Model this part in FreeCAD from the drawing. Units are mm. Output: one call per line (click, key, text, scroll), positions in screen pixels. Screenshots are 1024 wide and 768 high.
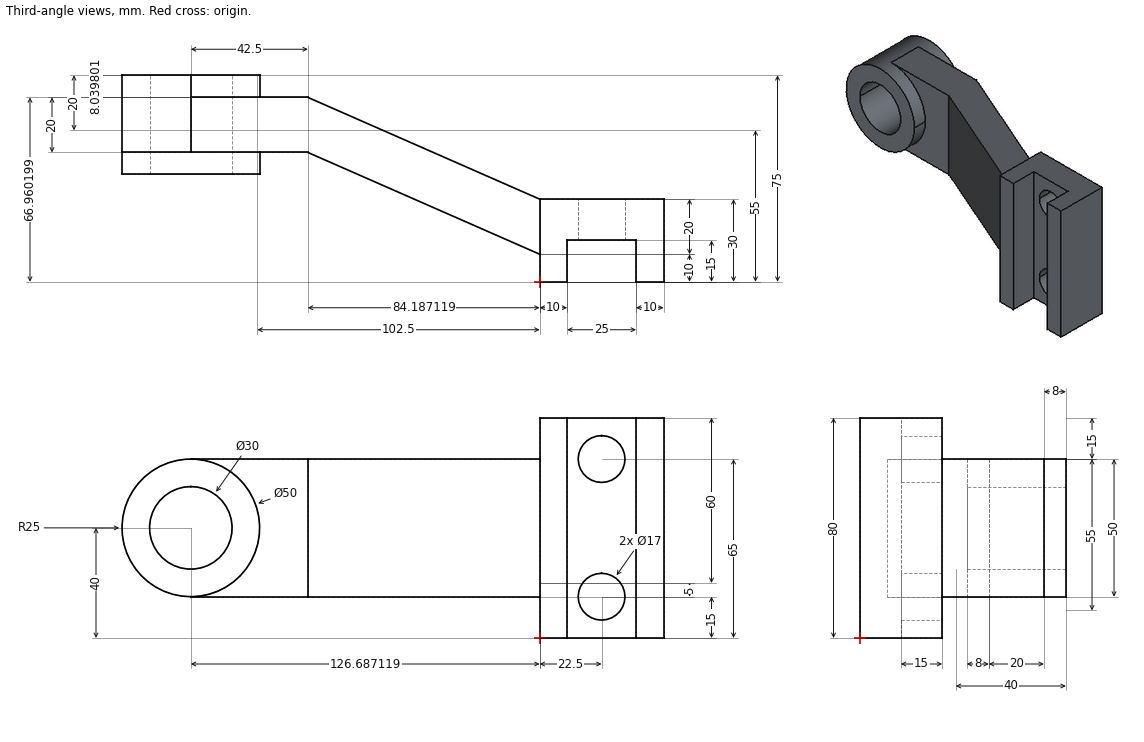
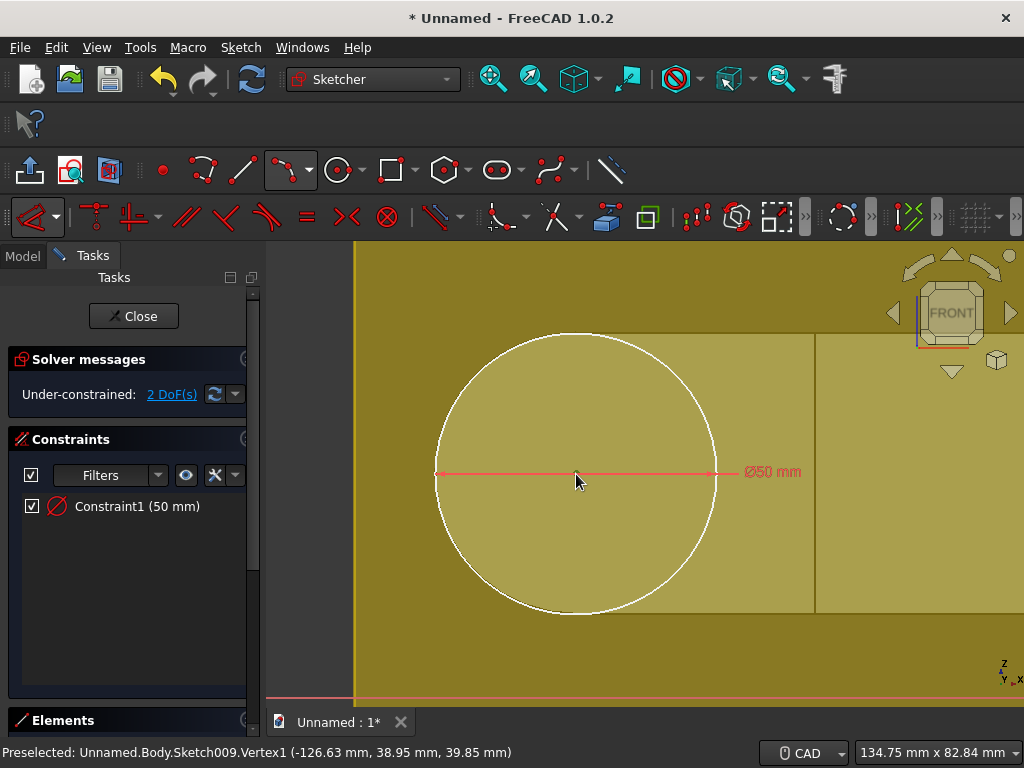
key(i)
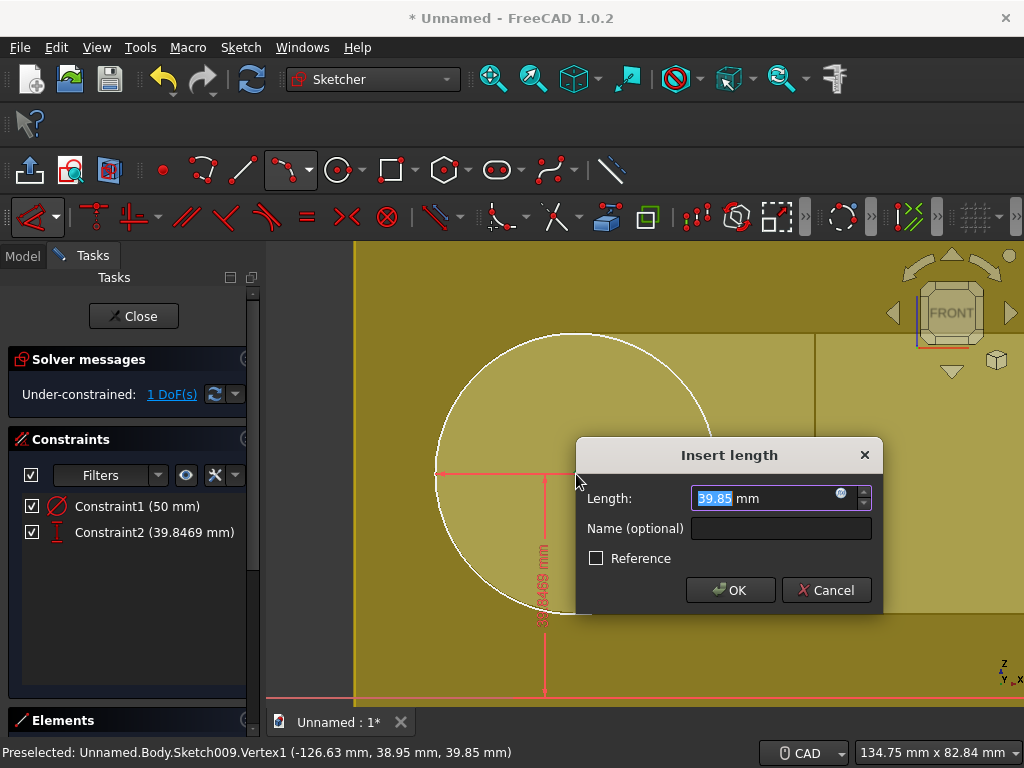
text(40)
key(Return)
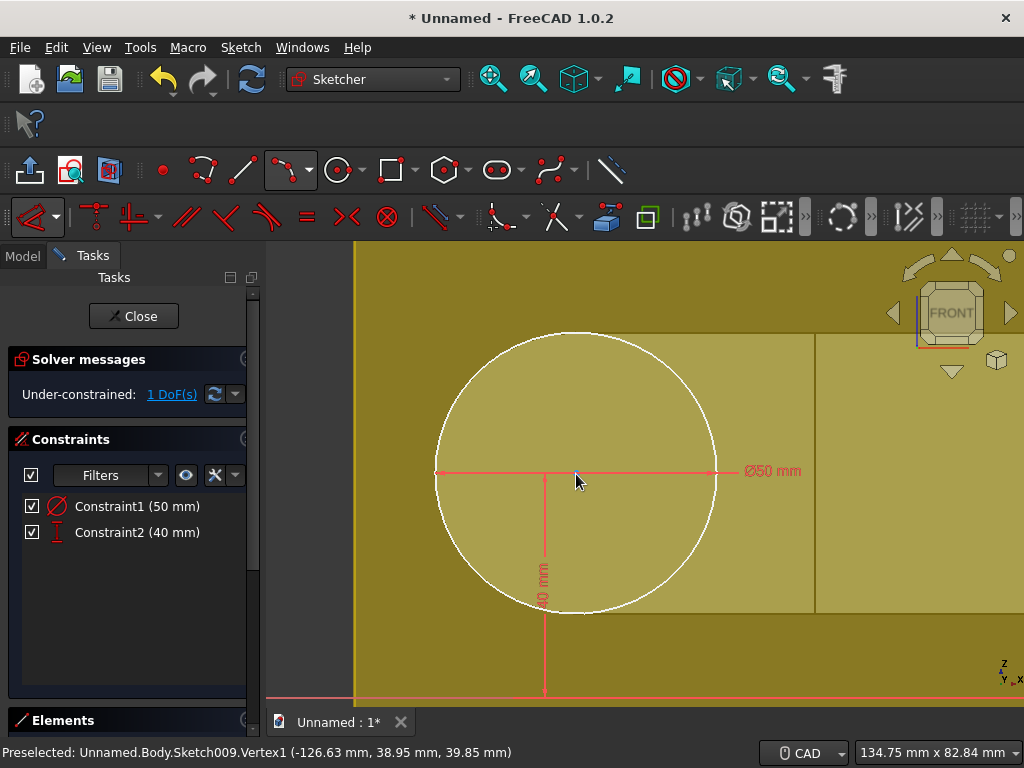
click(576, 473)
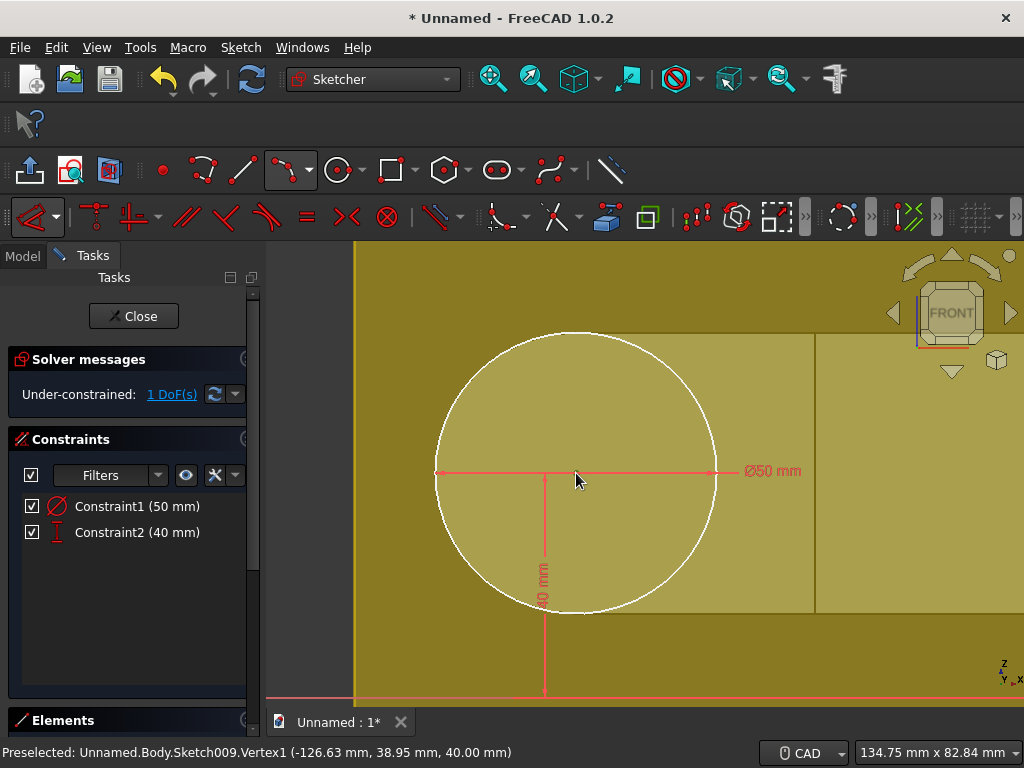
key(l)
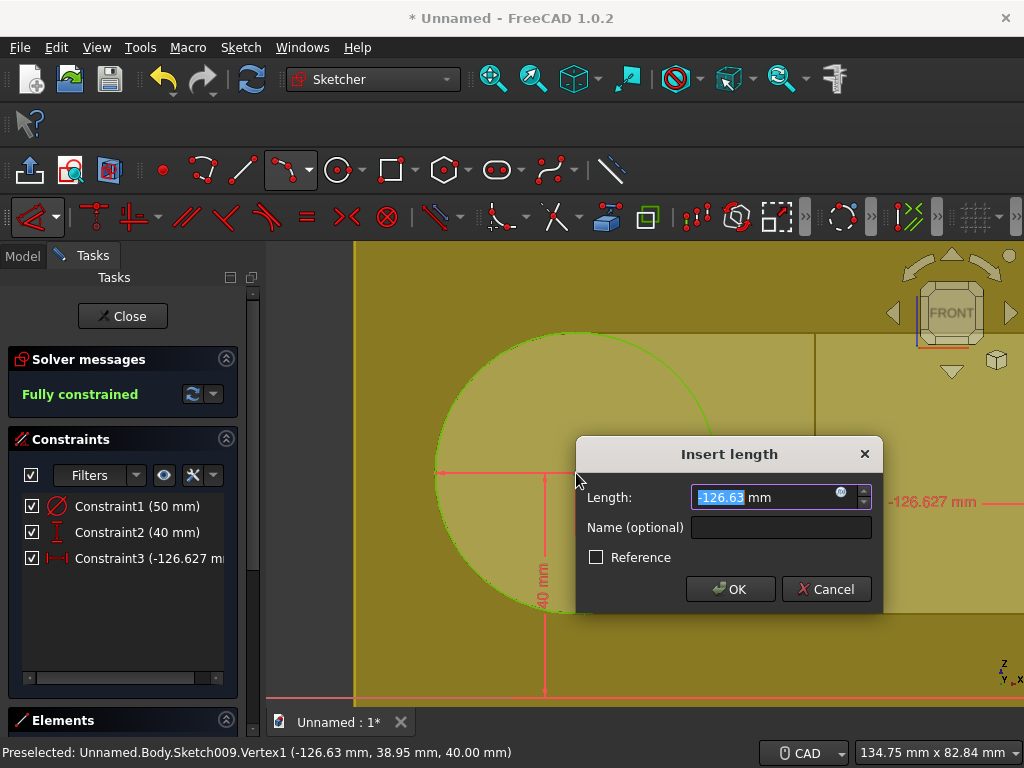
text(-126.687119)
key(Return)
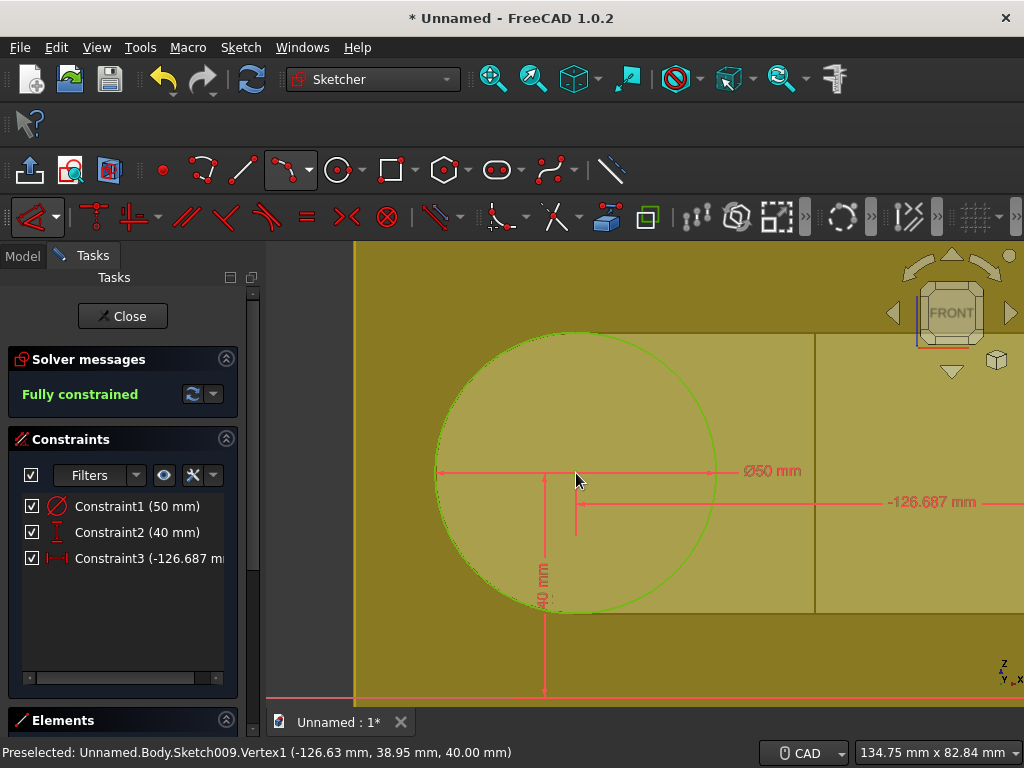
click(123, 316)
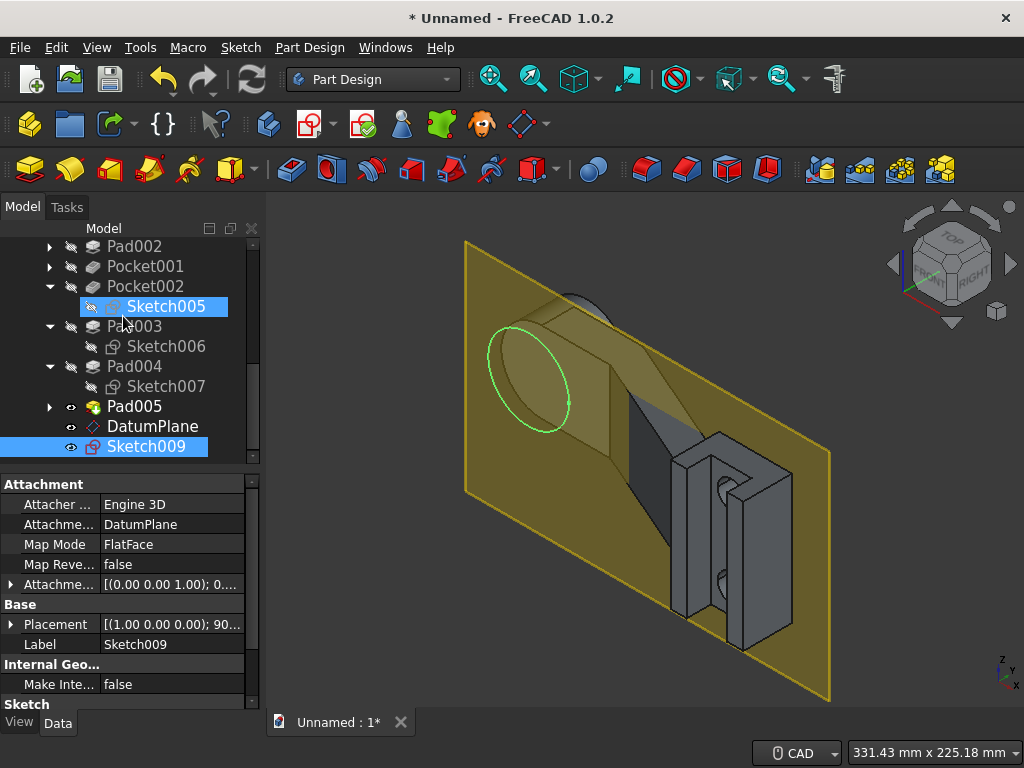
click(30, 170)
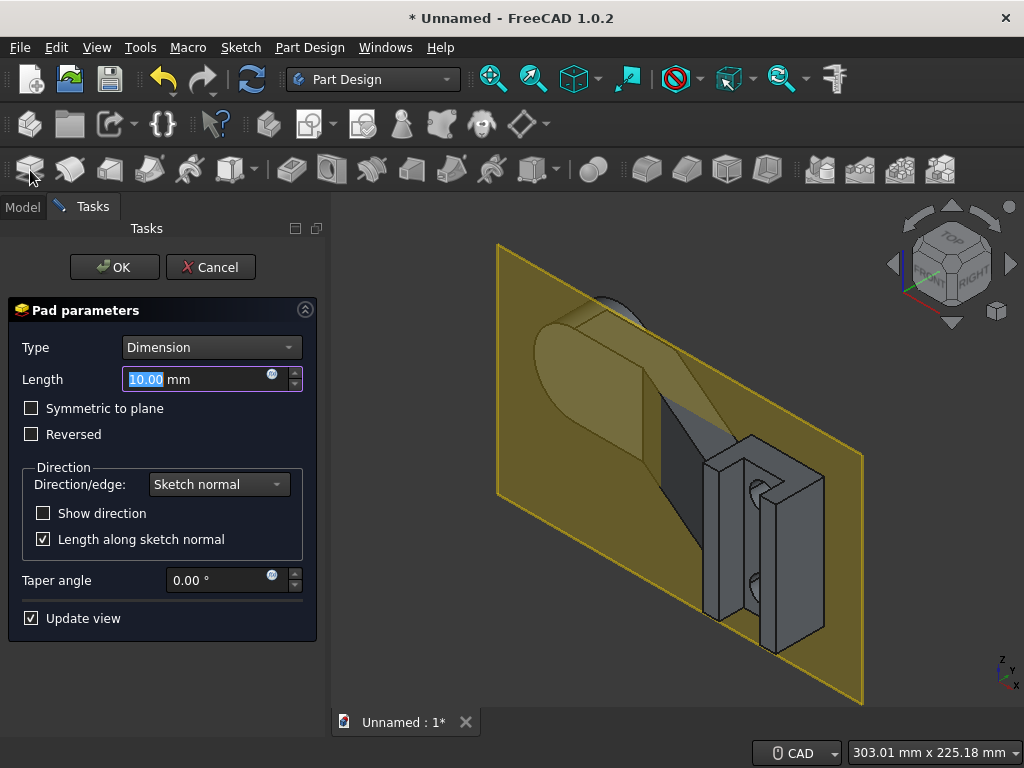
text(8)
key(Tab)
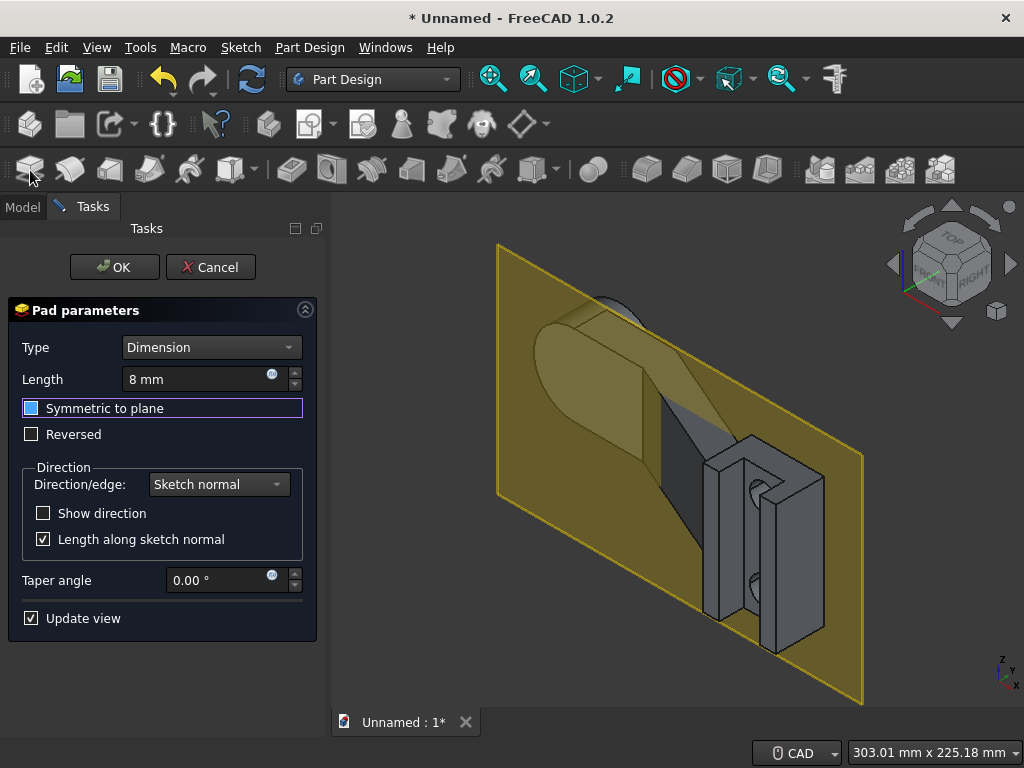
click(30, 434)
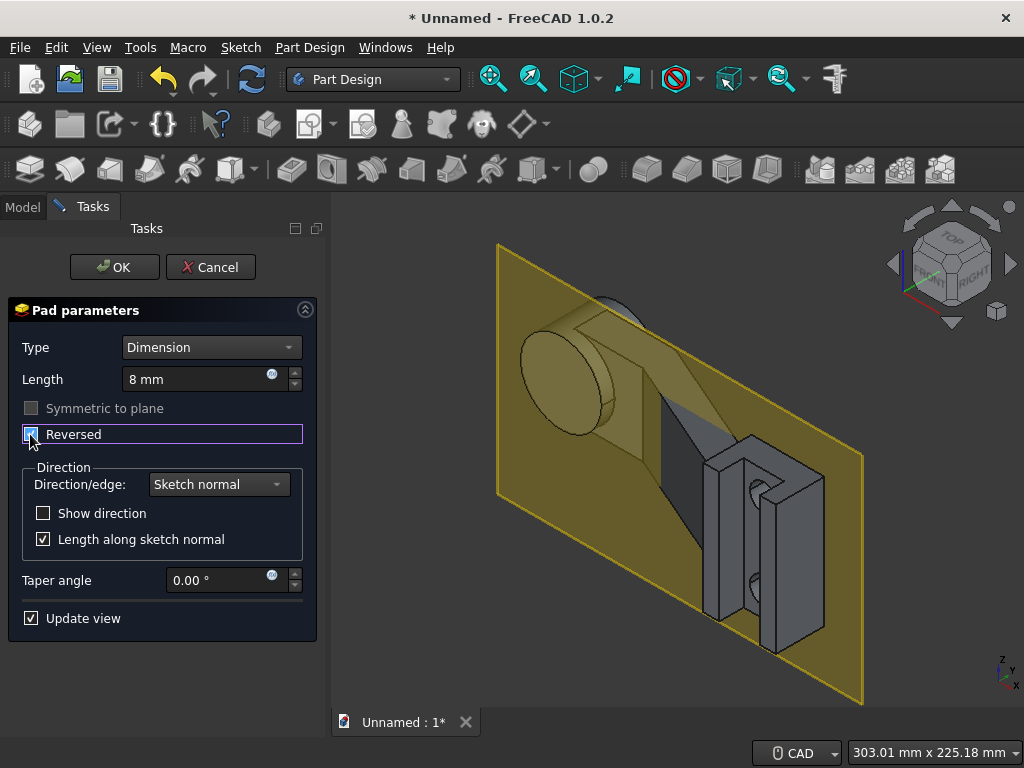
click(115, 267)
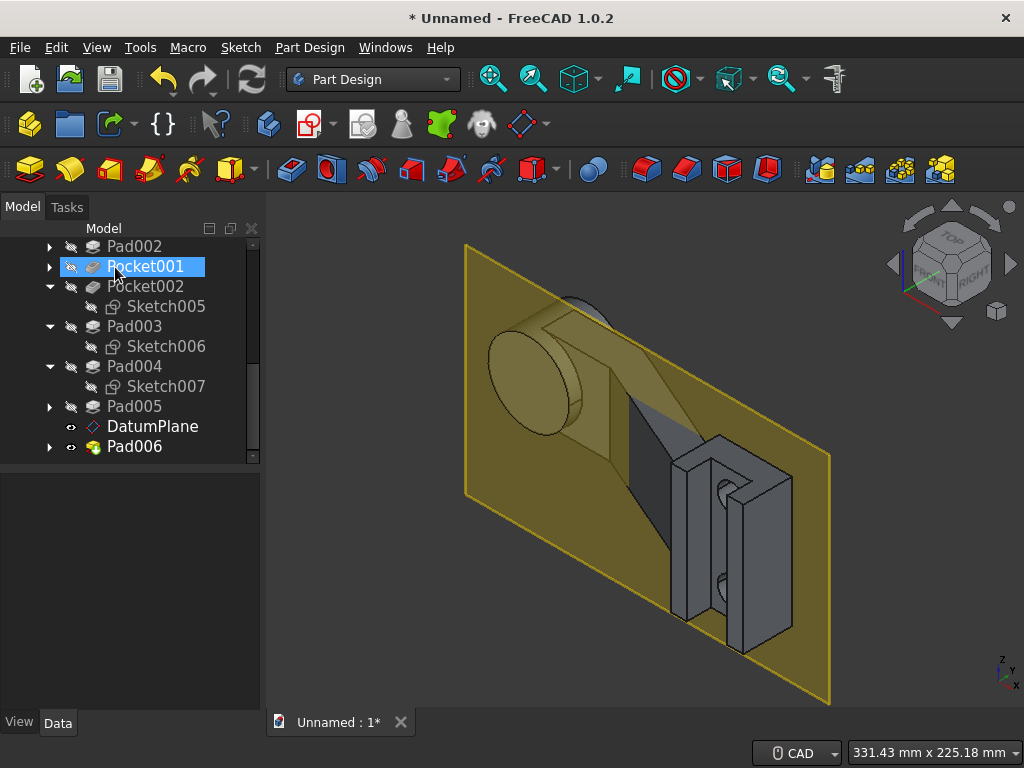
click(116, 427)
key(space)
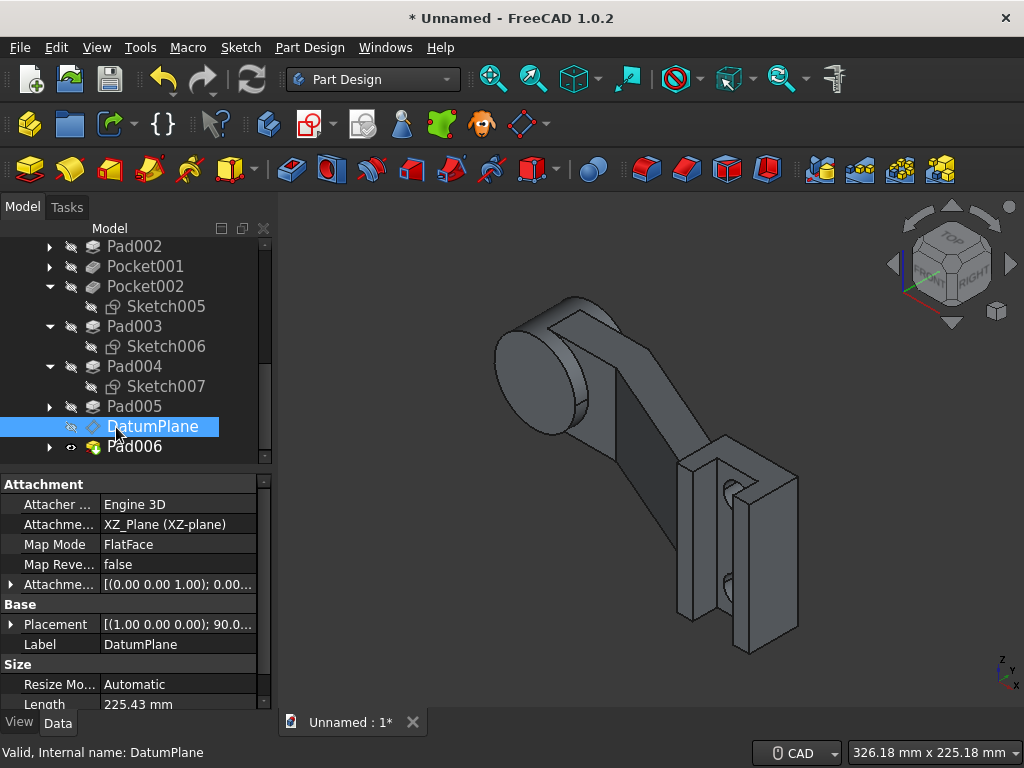
key(4)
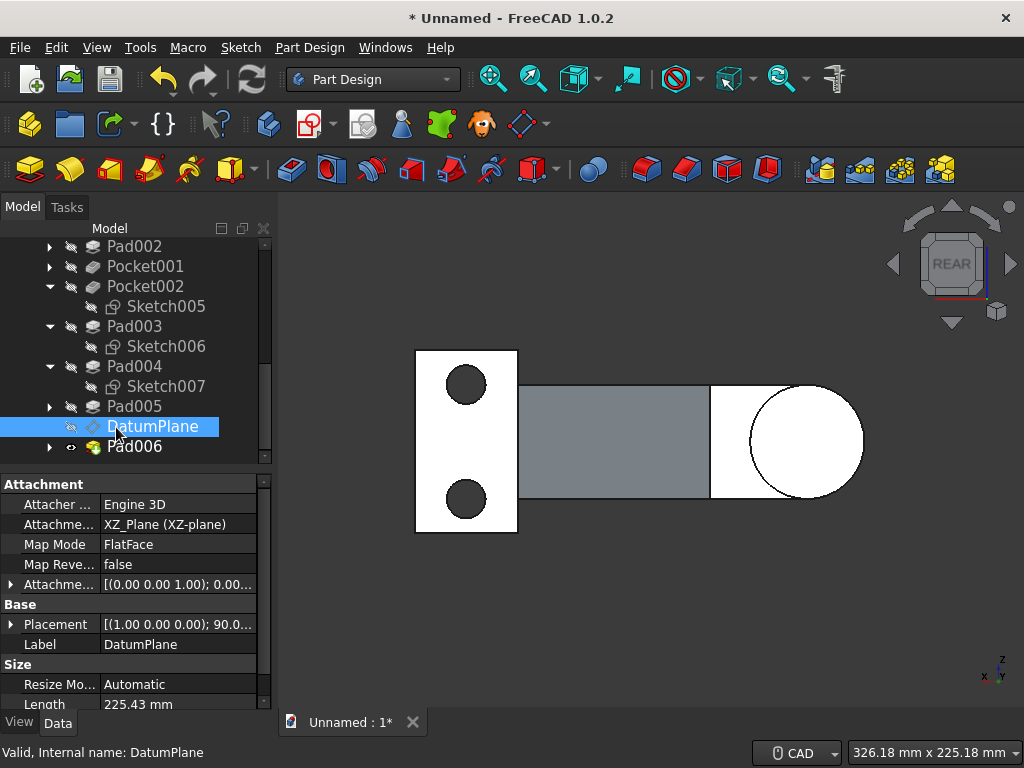
click(807, 441)